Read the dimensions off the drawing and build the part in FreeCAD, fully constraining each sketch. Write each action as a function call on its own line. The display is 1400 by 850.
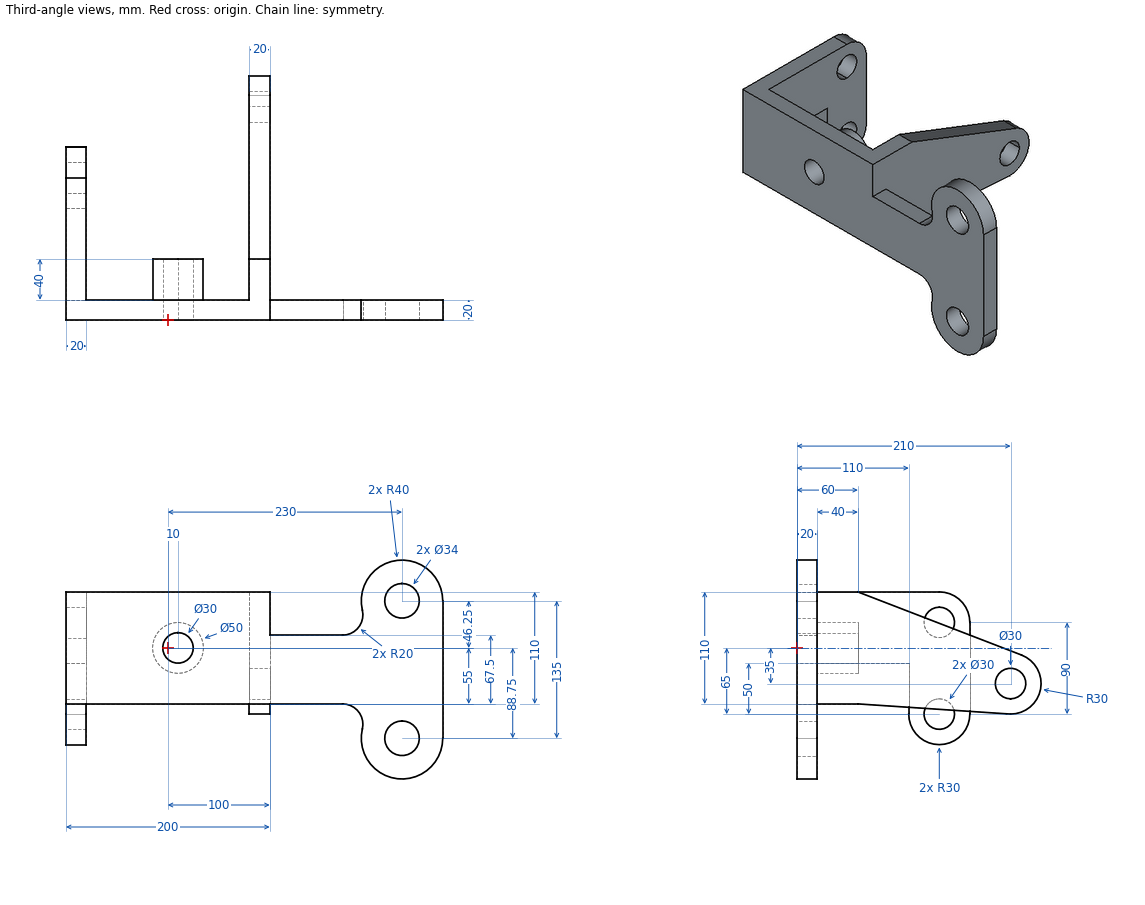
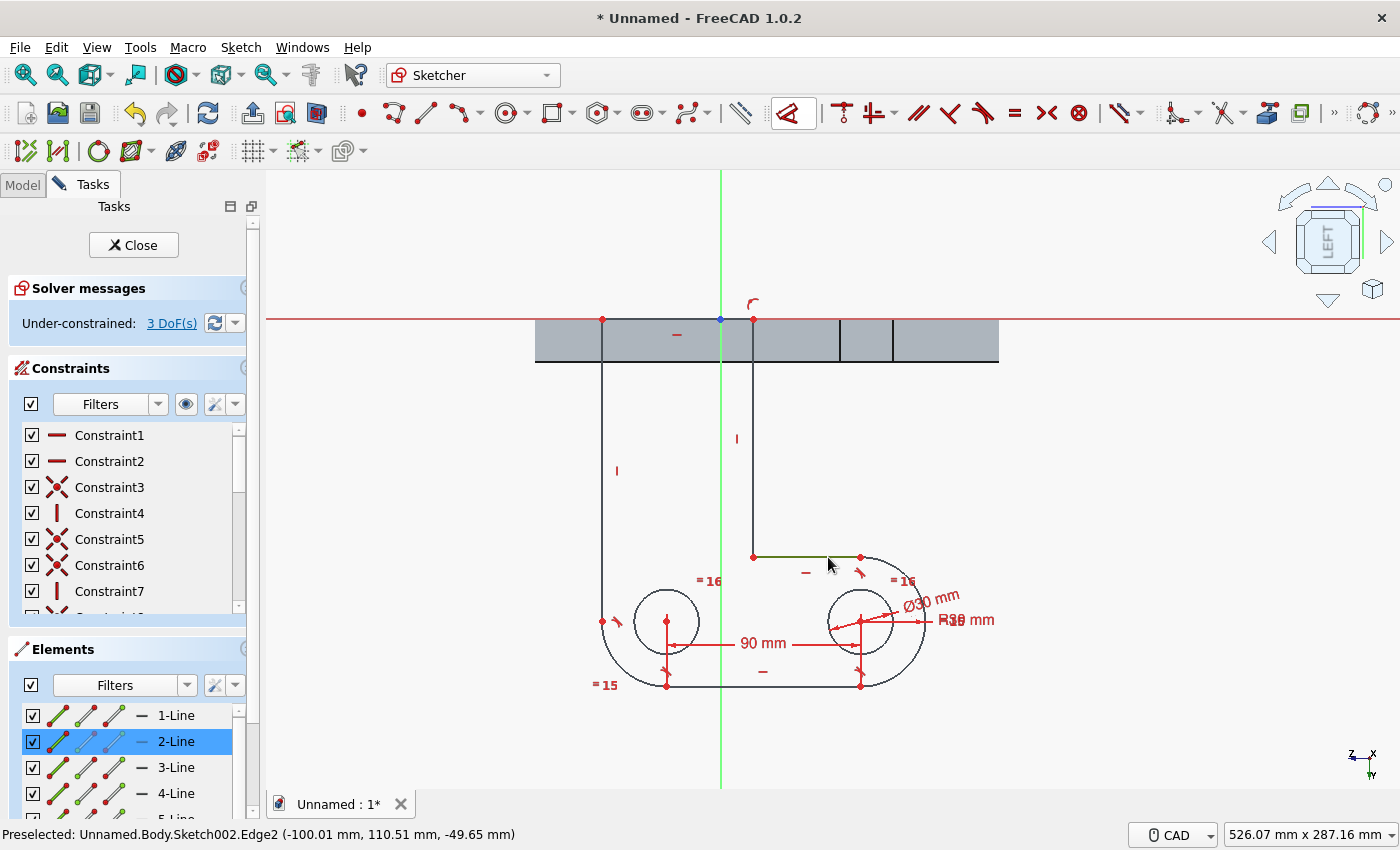
key(l)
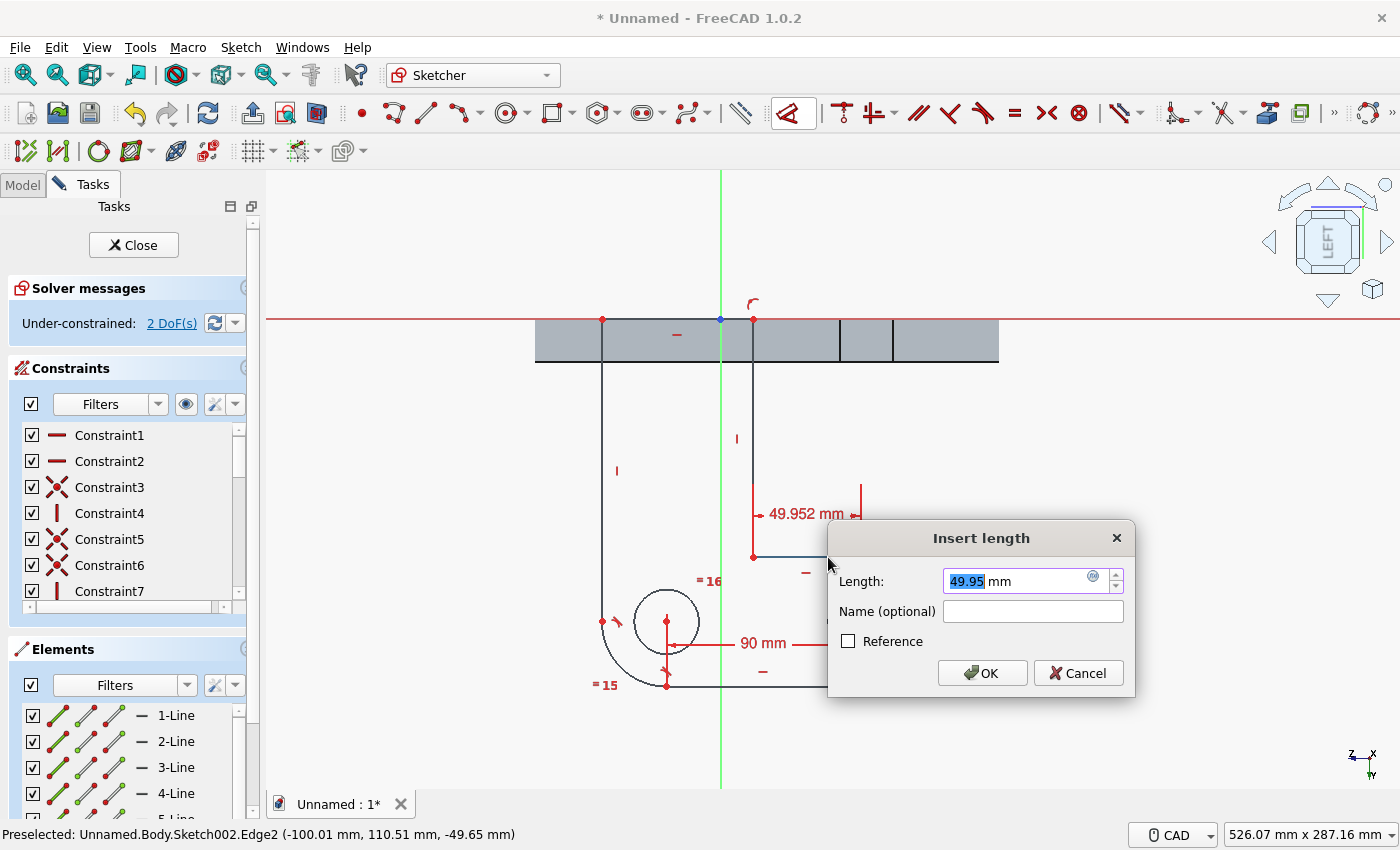
text(50)
key(Return)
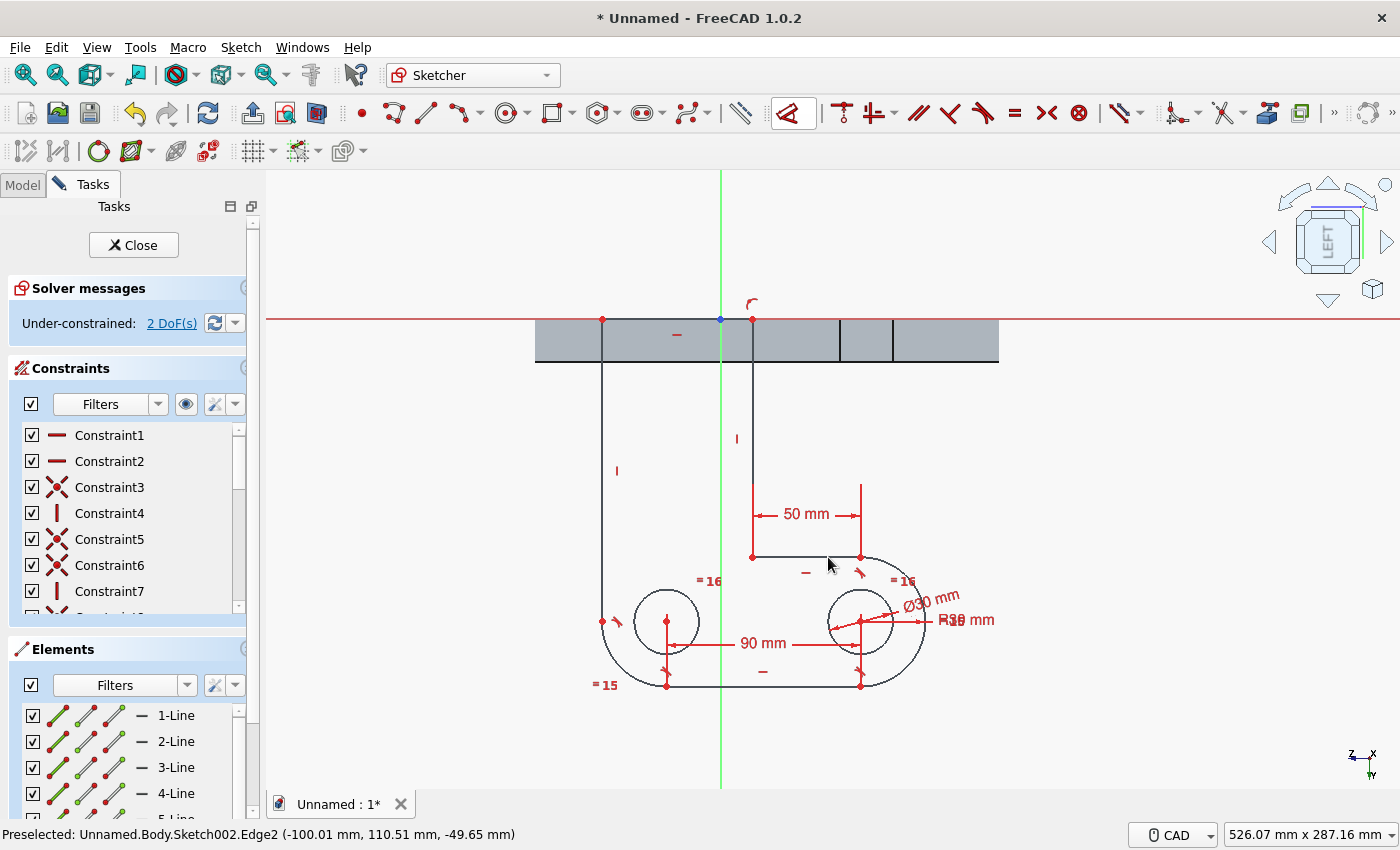
click(861, 622)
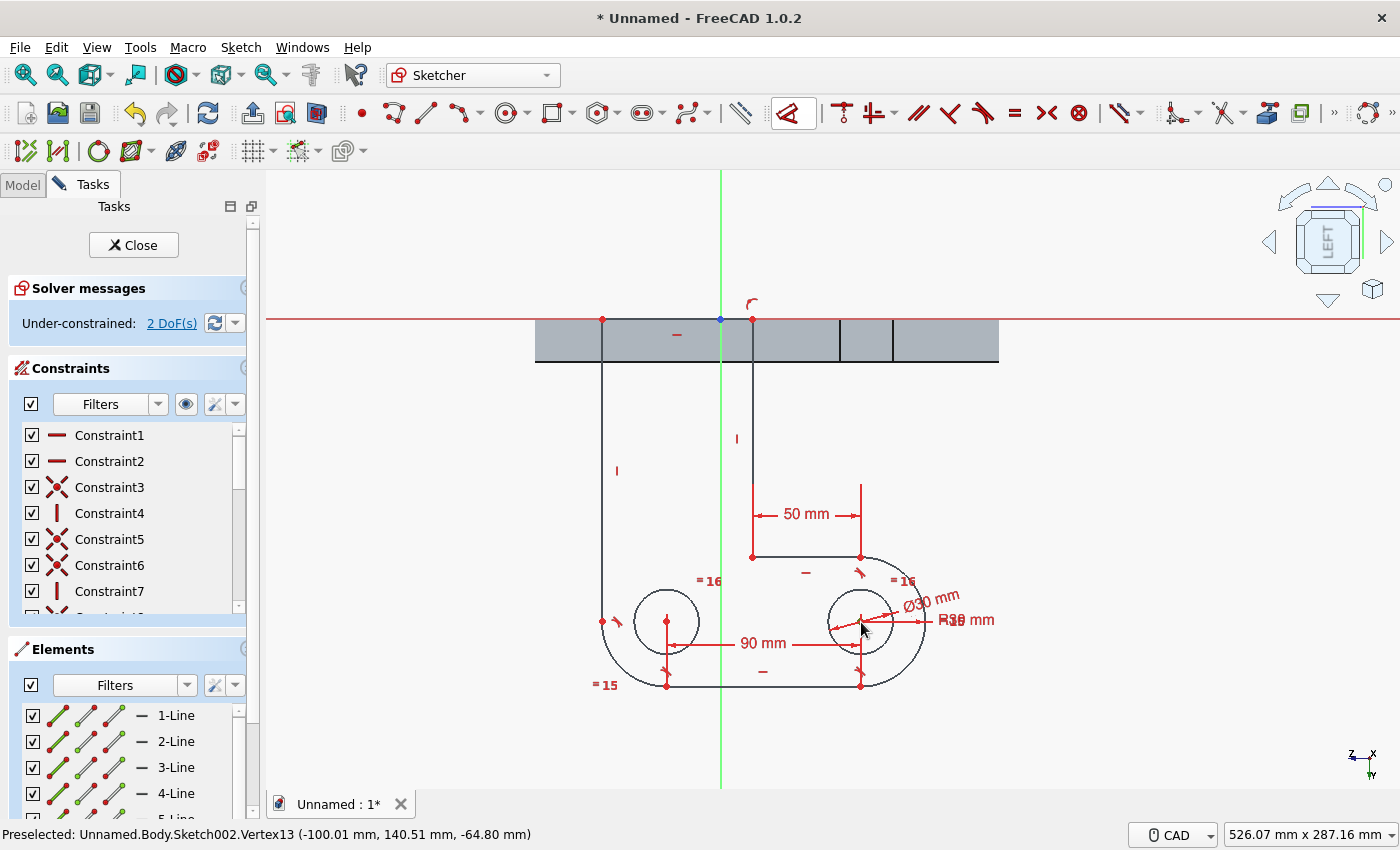
click(810, 114)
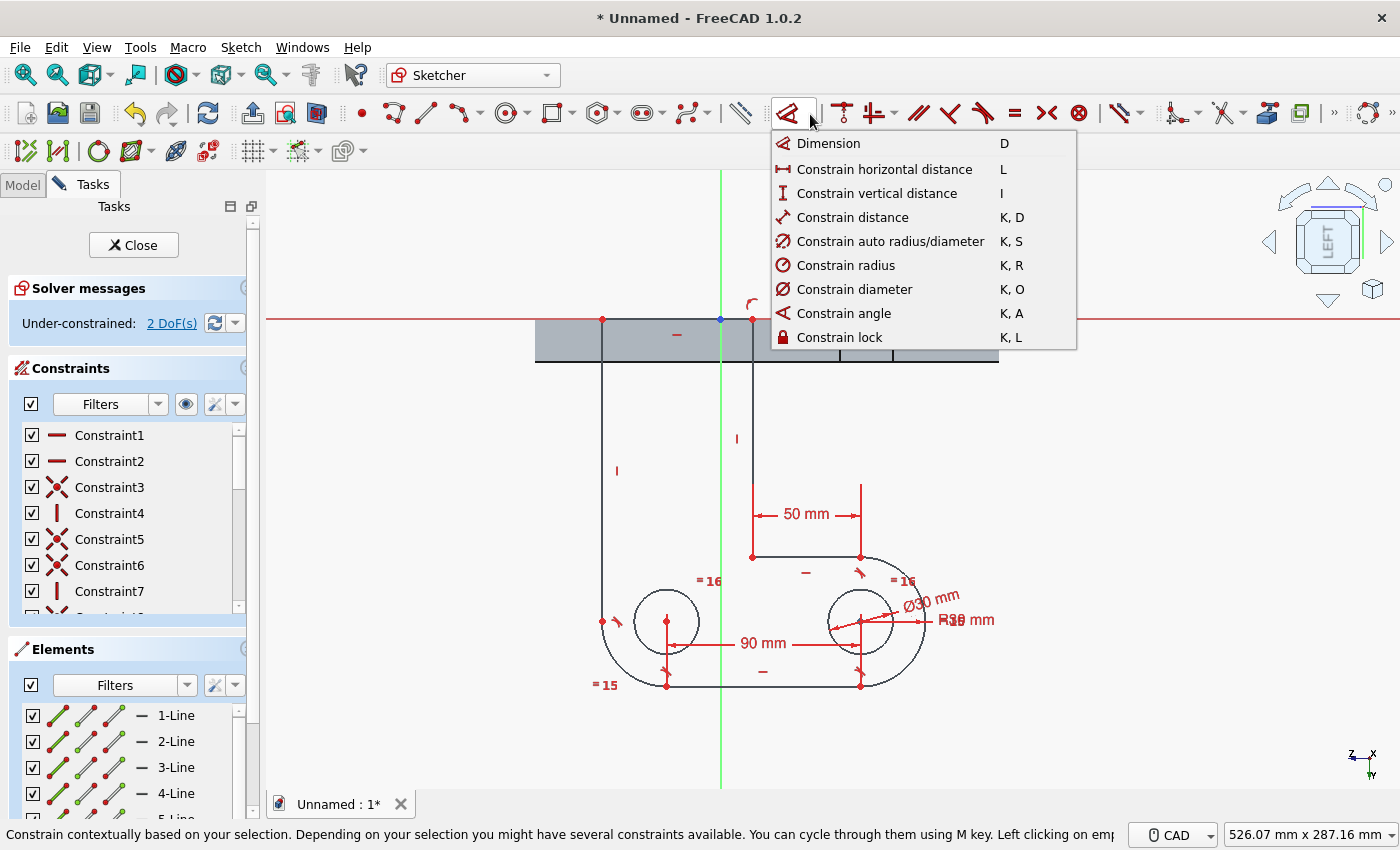
click(924, 169)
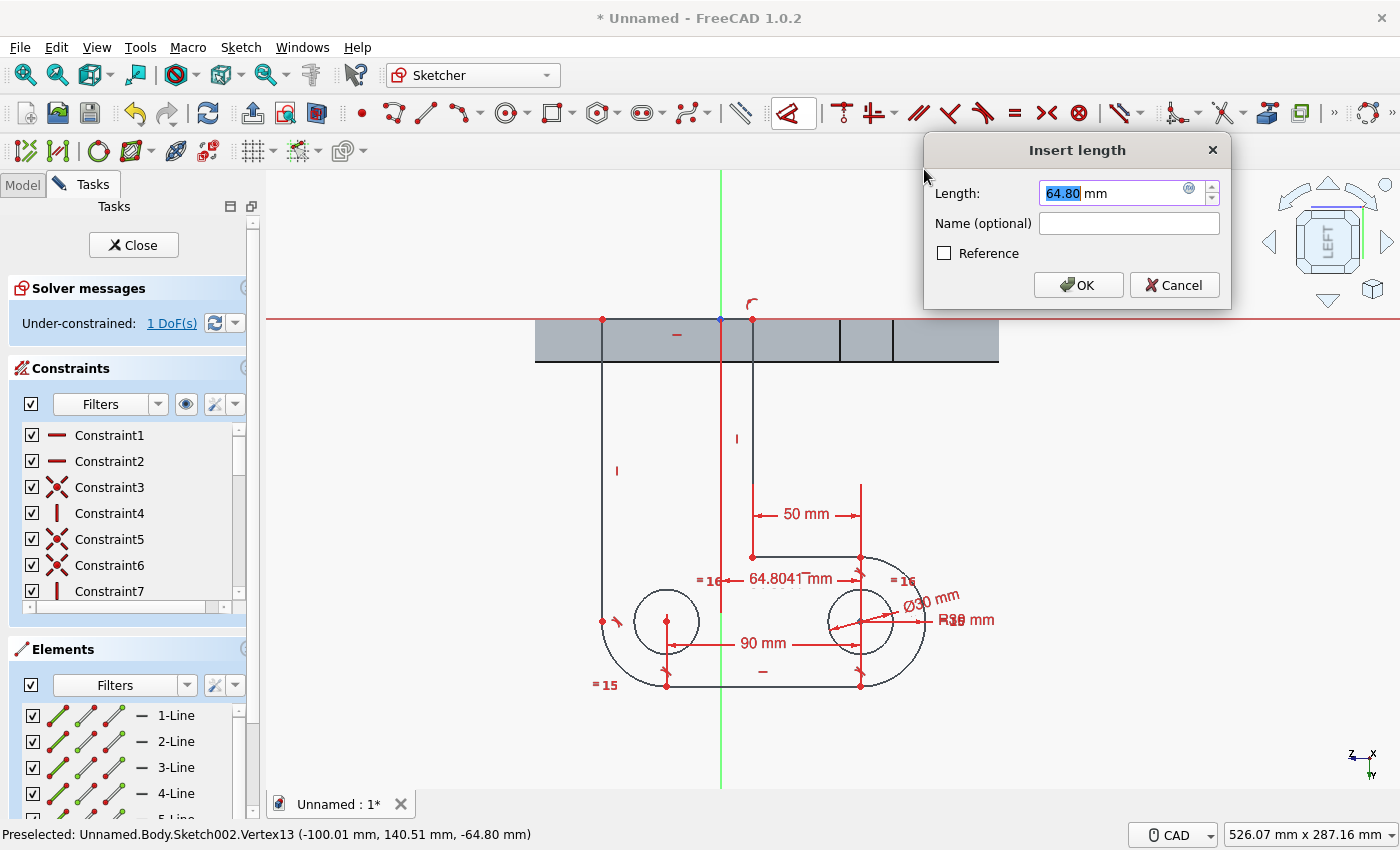
text(65)
key(Return)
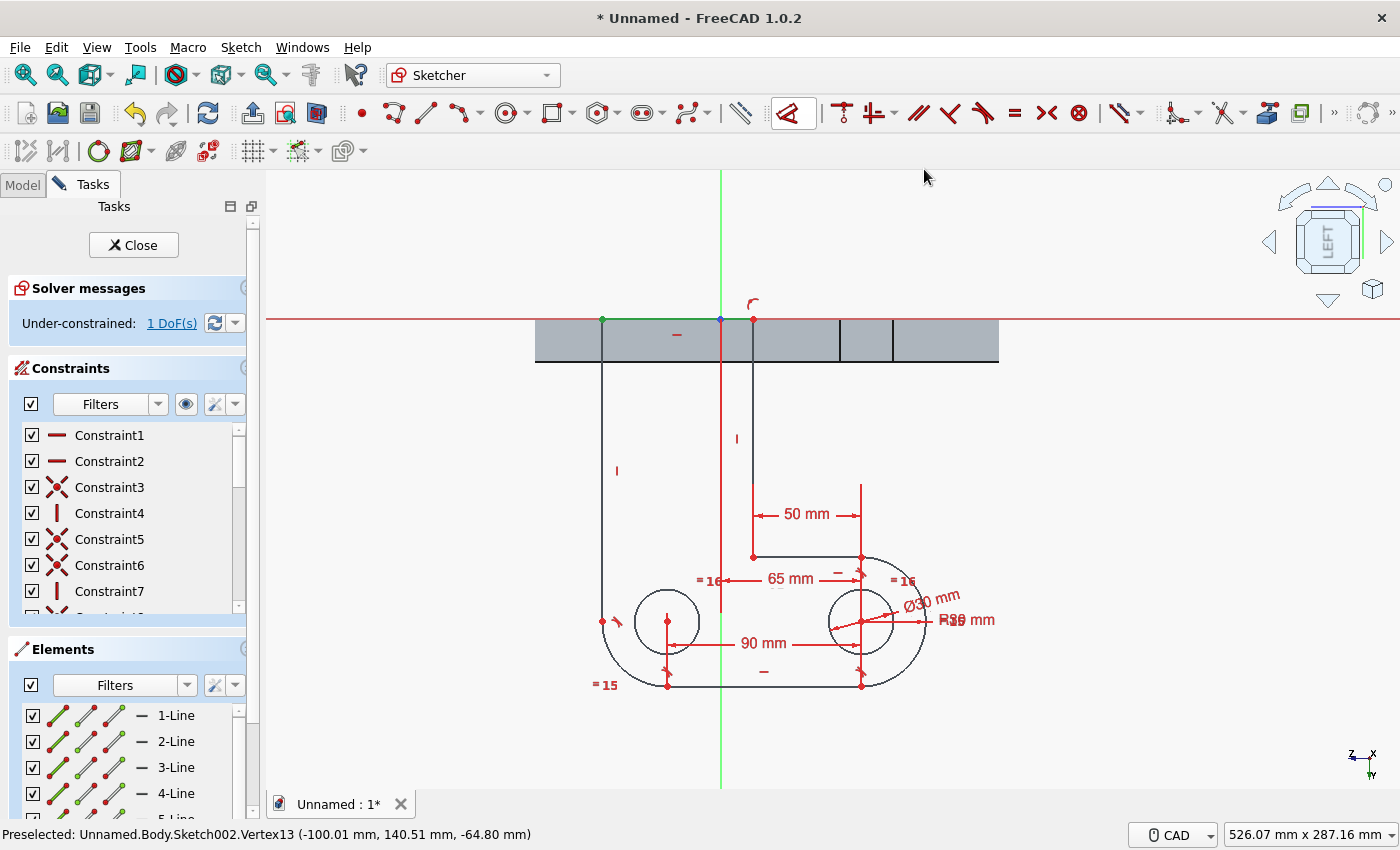
click(753, 486)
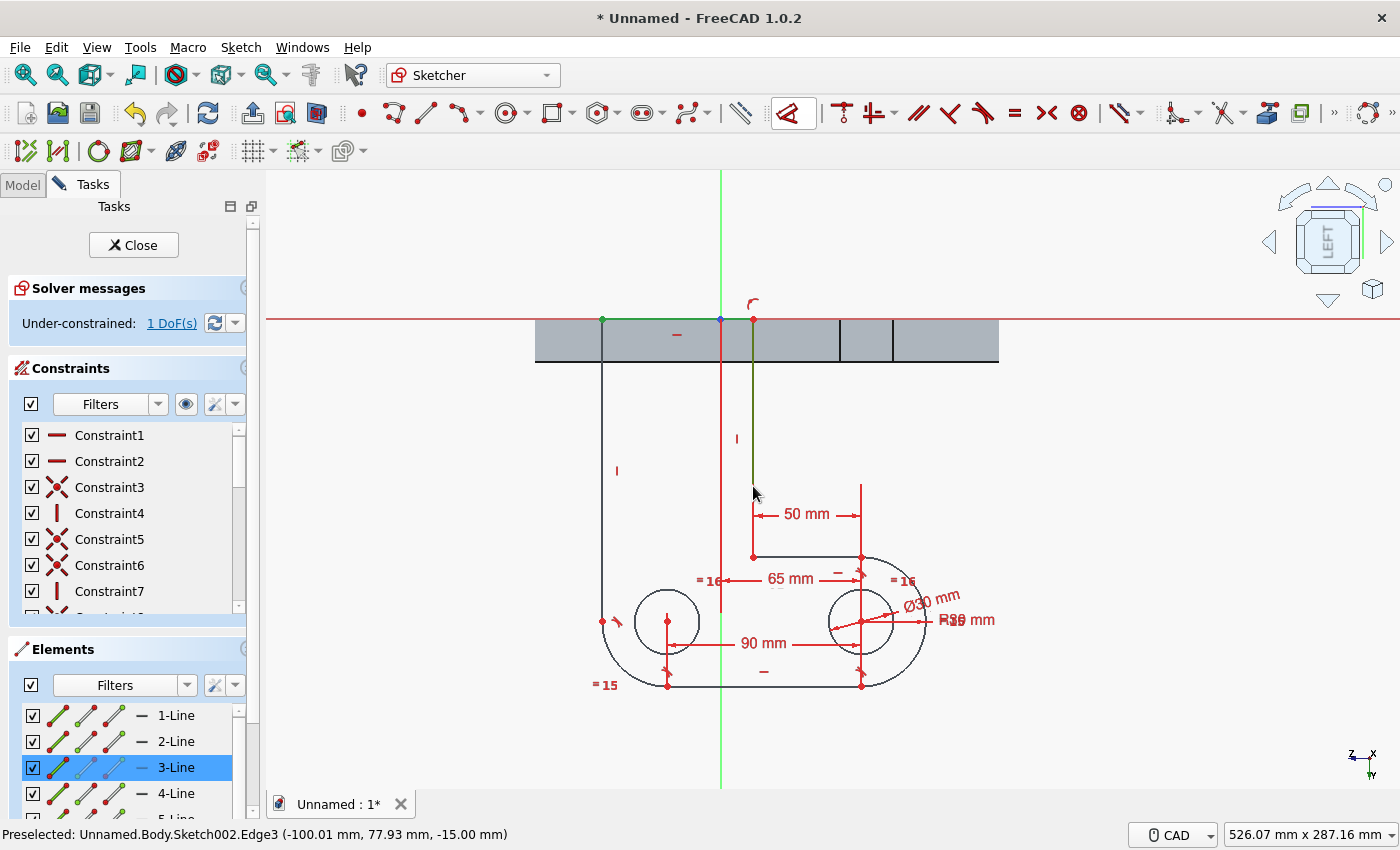
key(i)